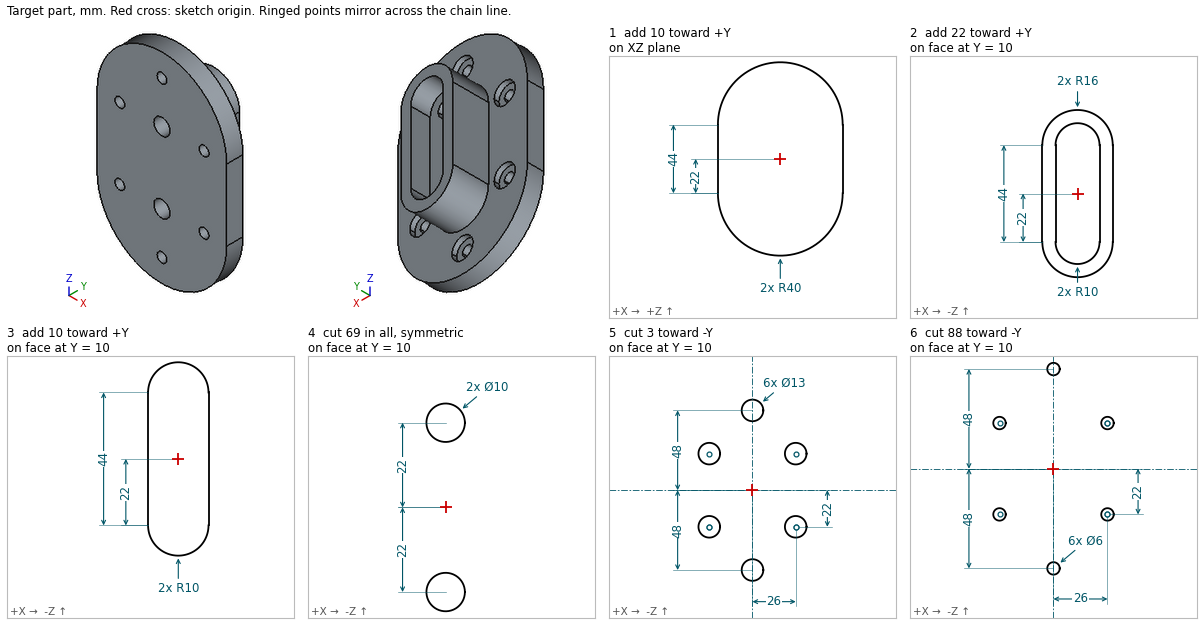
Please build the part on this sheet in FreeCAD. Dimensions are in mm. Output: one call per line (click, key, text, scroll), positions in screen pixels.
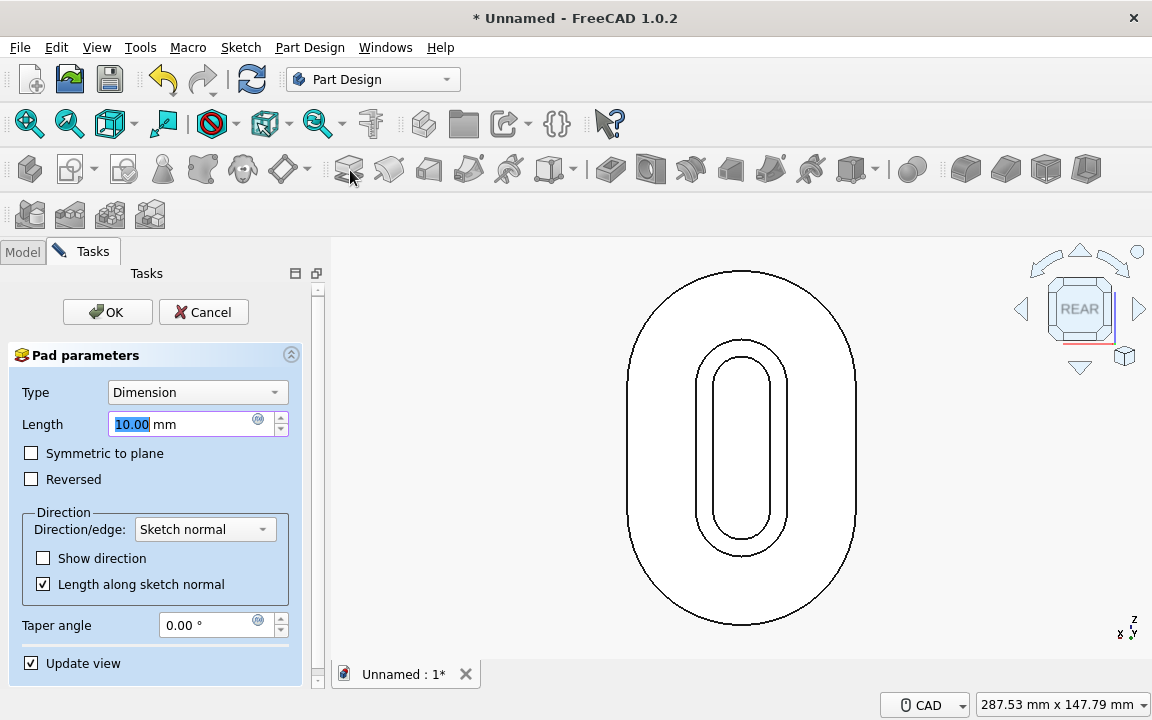
text(10)
key(Tab)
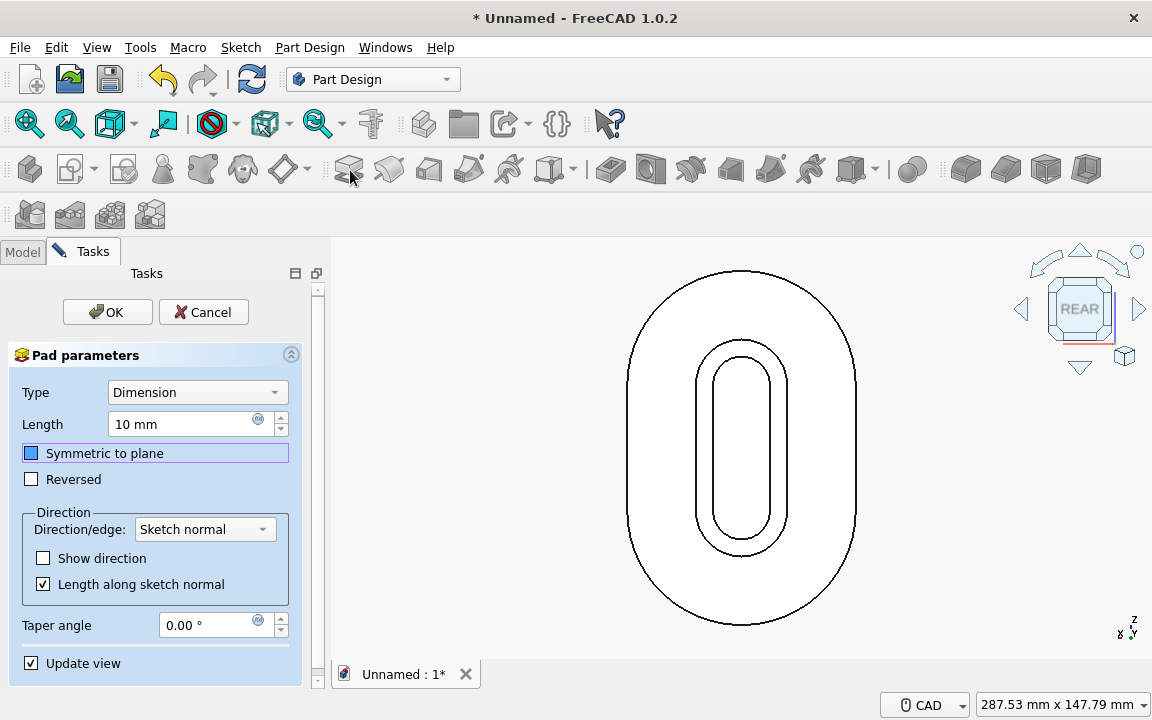
click(108, 312)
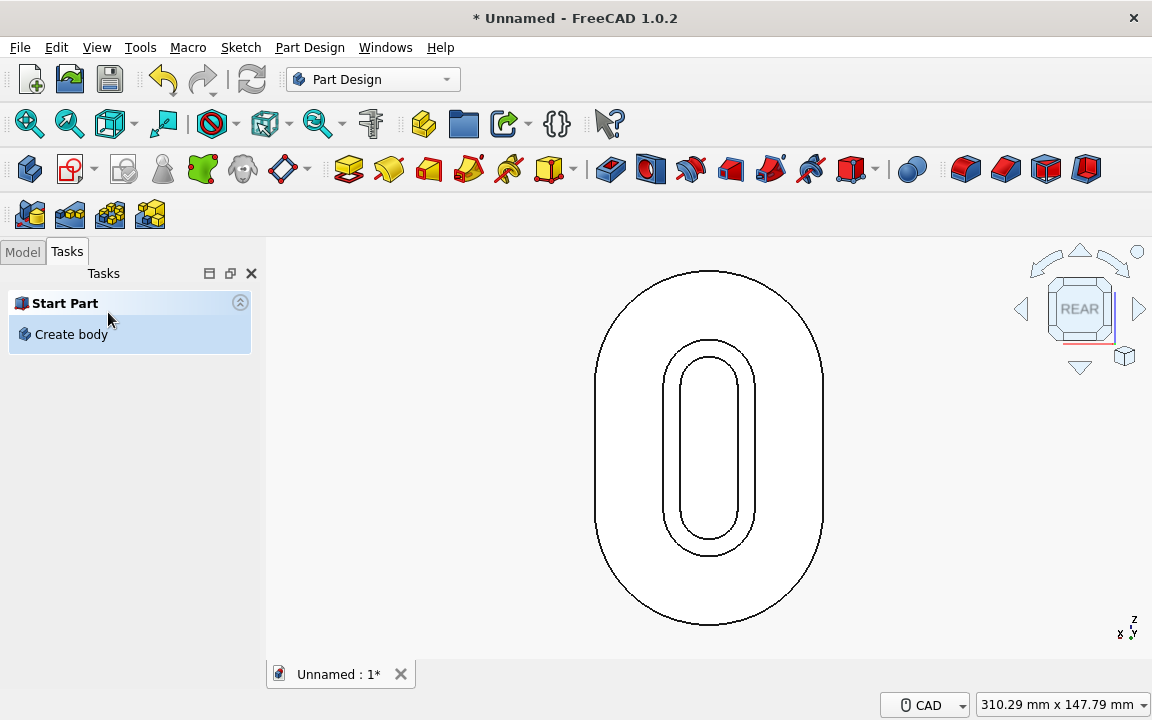
click(644, 548)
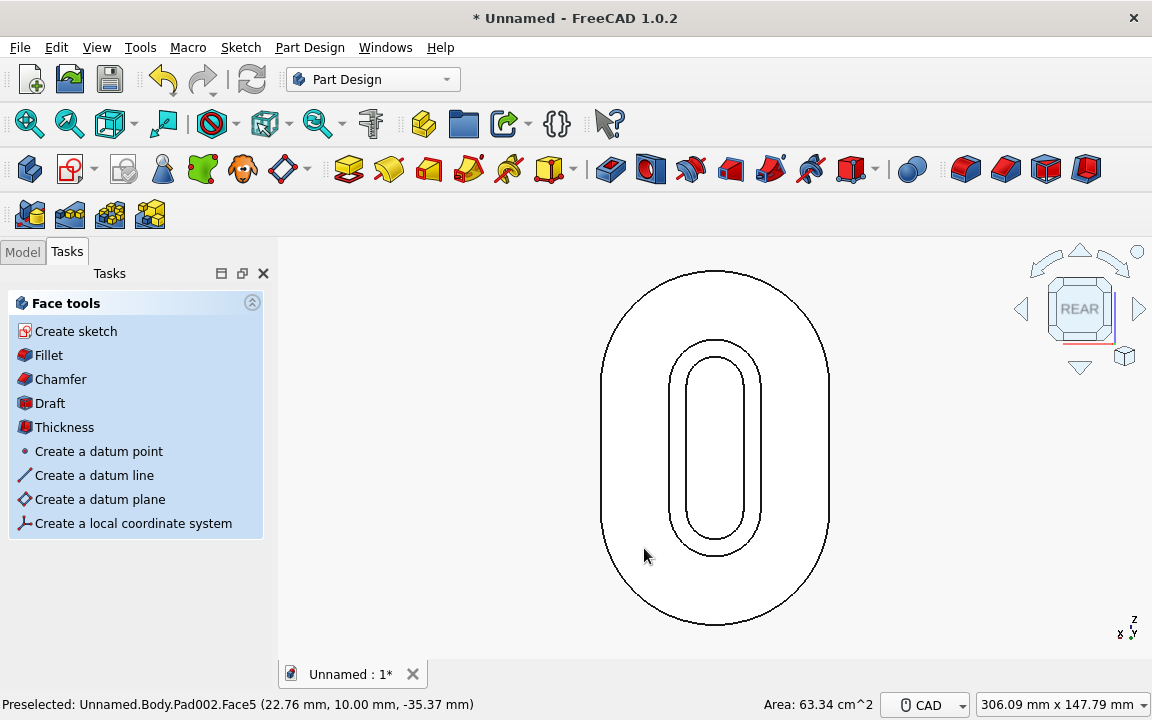
click(70, 170)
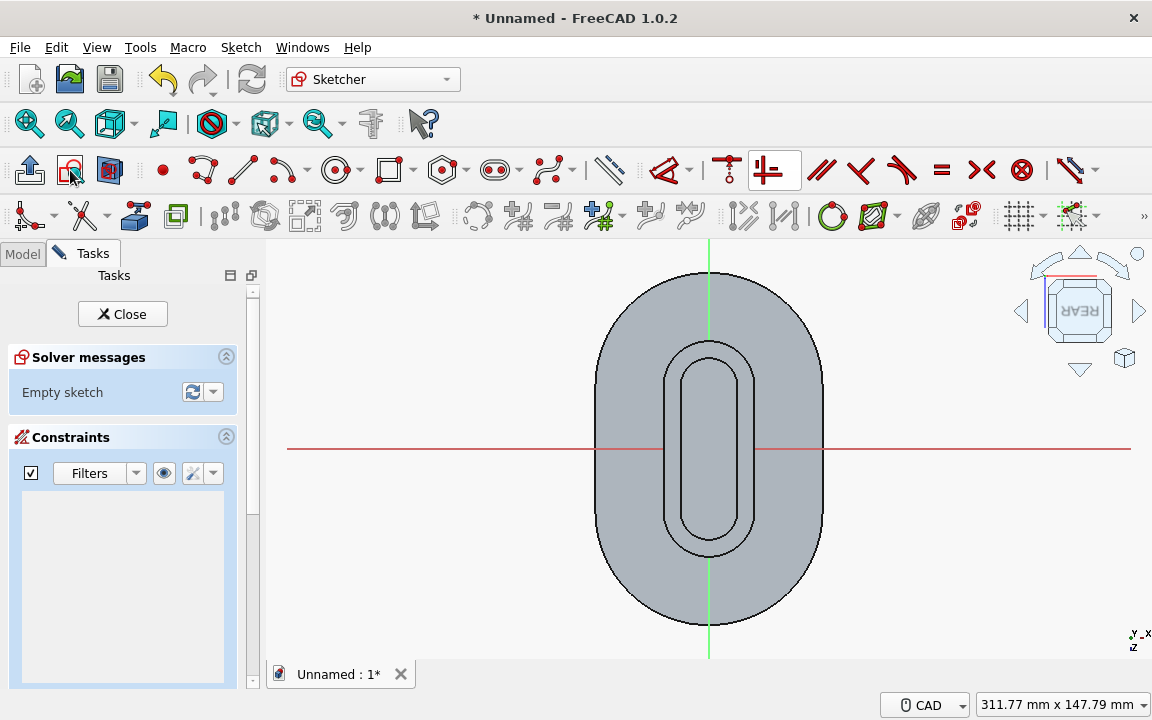
scroll(792, 449, up, 3)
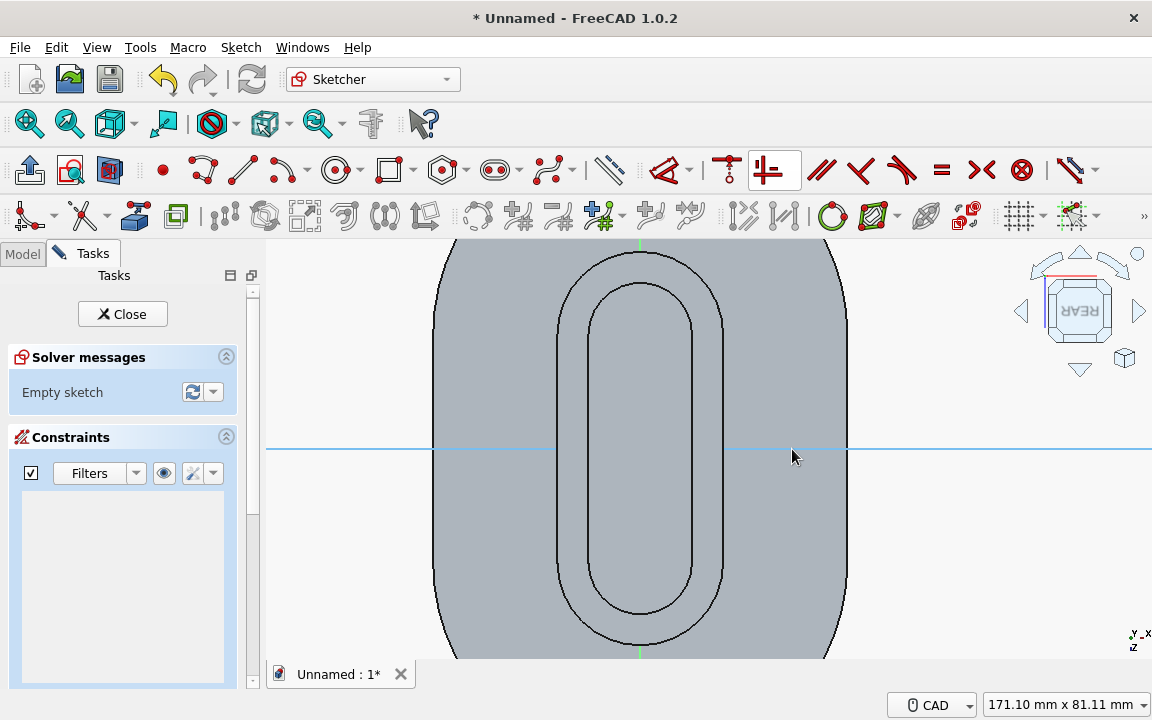
click(336, 170)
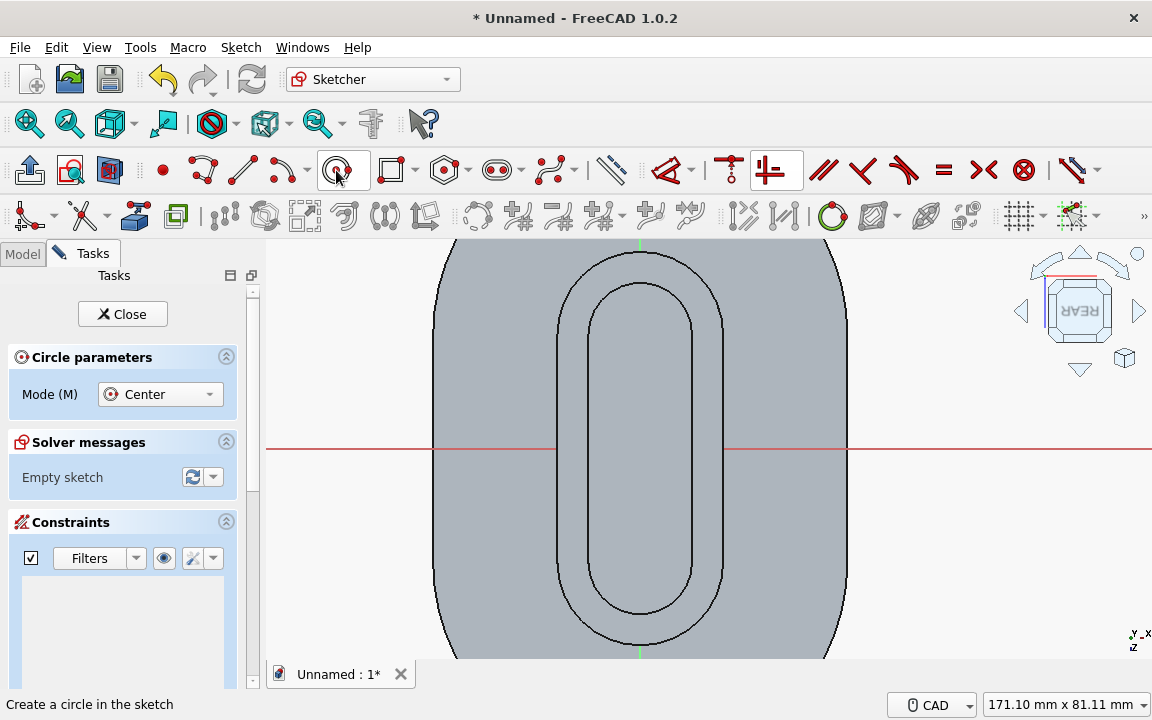
click(640, 335)
move(659, 316)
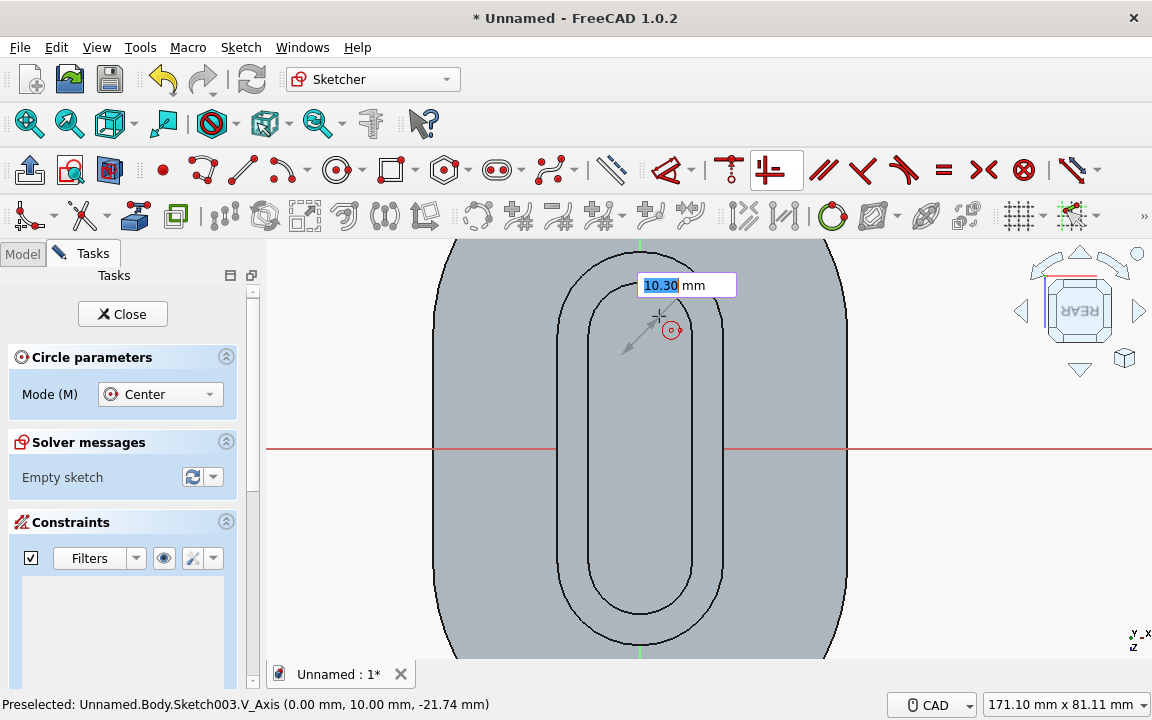
text(10)
key(Return)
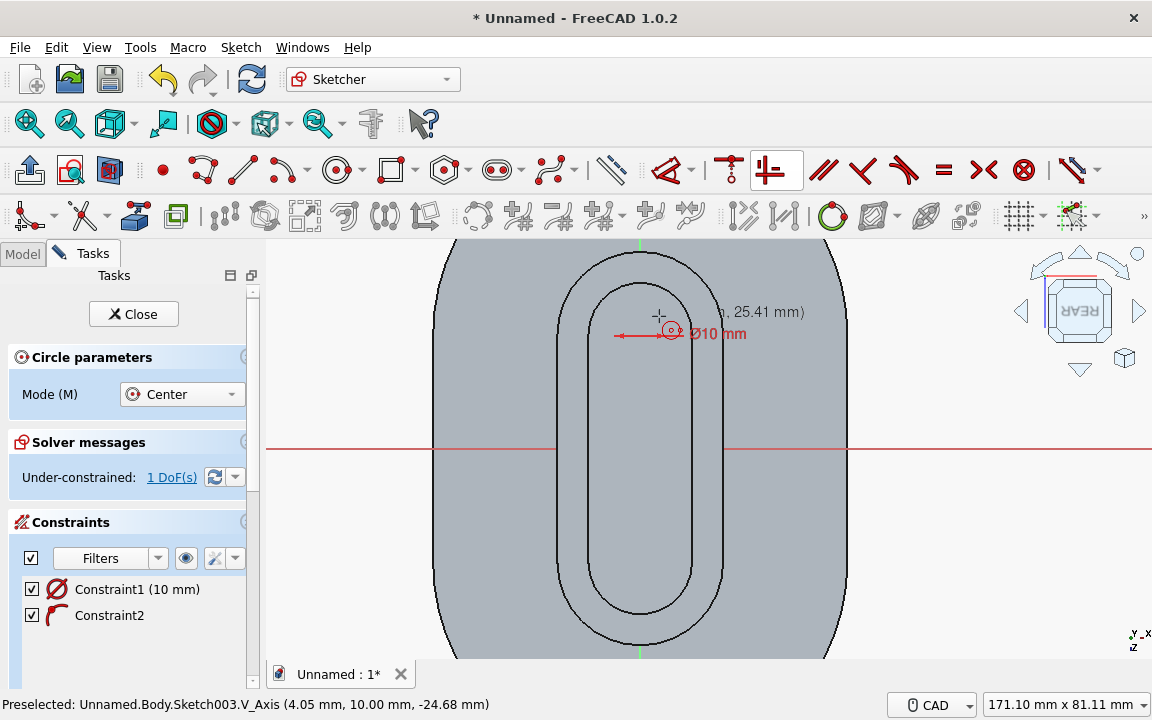
click(640, 563)
move(659, 544)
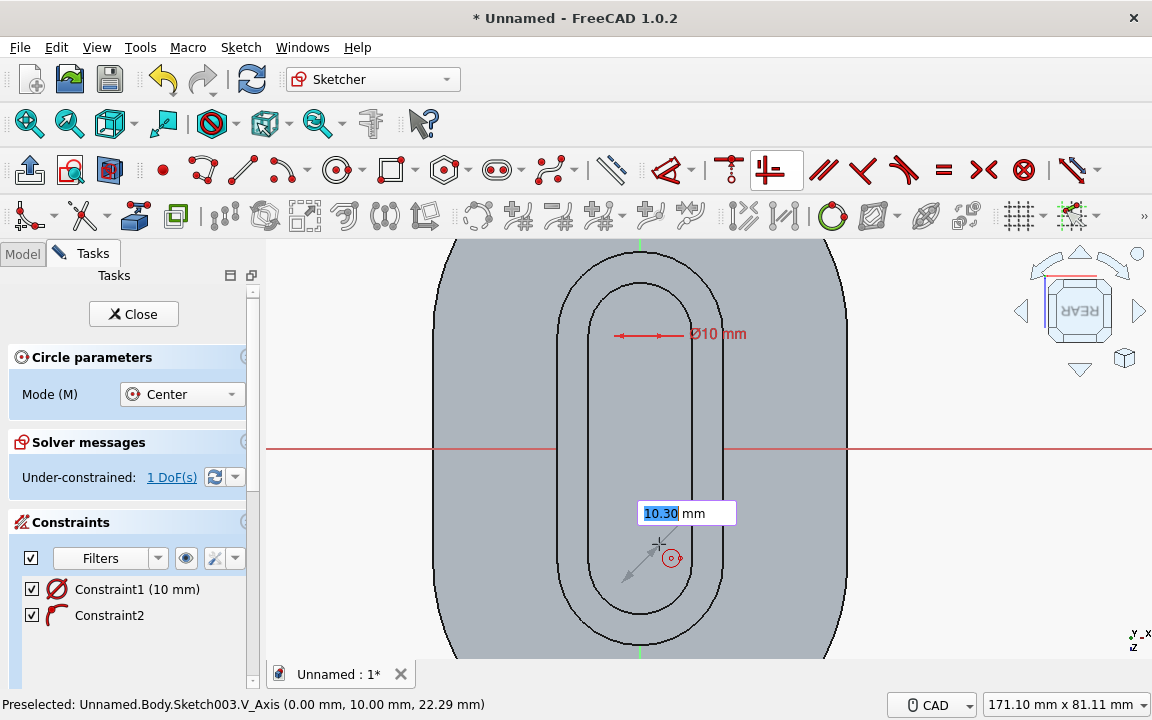
text(10)
key(Return)
key(Escape)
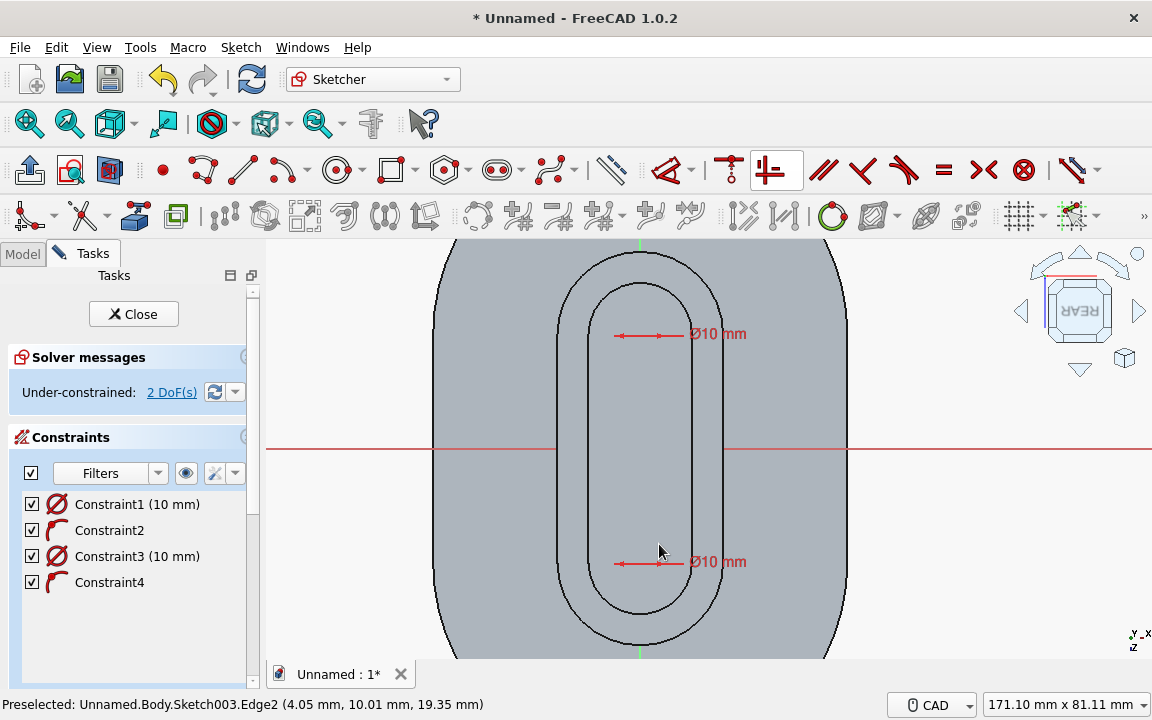
click(666, 170)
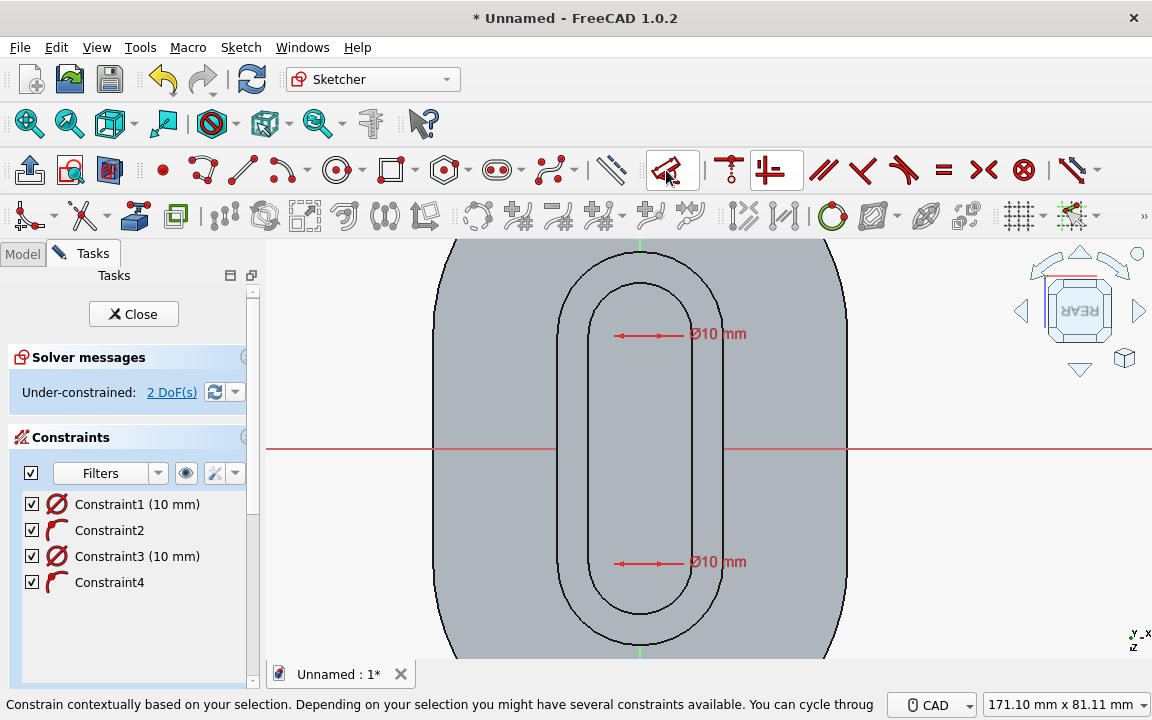
click(640, 336)
click(674, 392)